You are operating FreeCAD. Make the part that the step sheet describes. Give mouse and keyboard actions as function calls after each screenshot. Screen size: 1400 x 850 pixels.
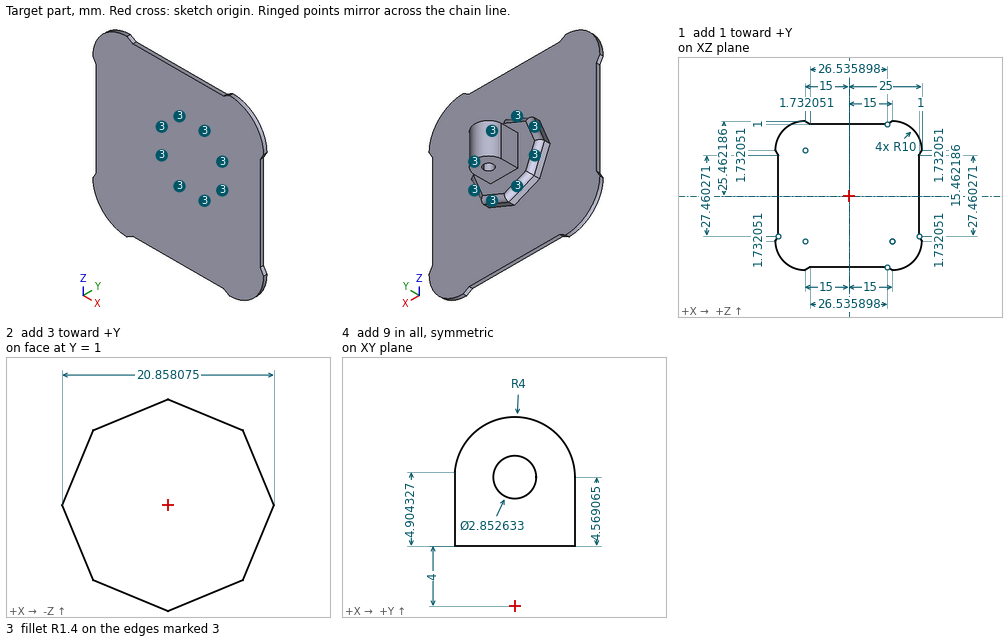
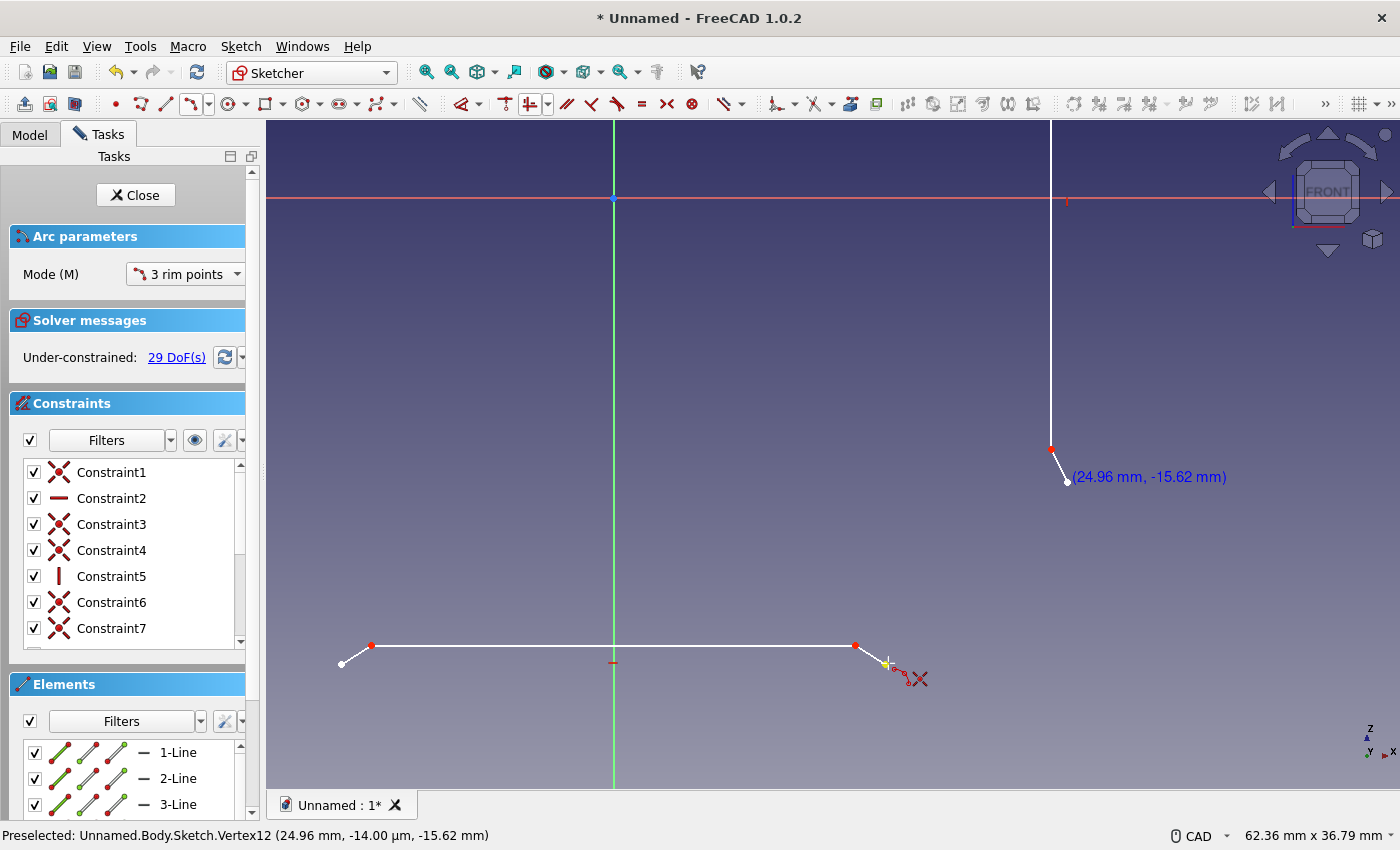
click(885, 665)
click(1015, 608)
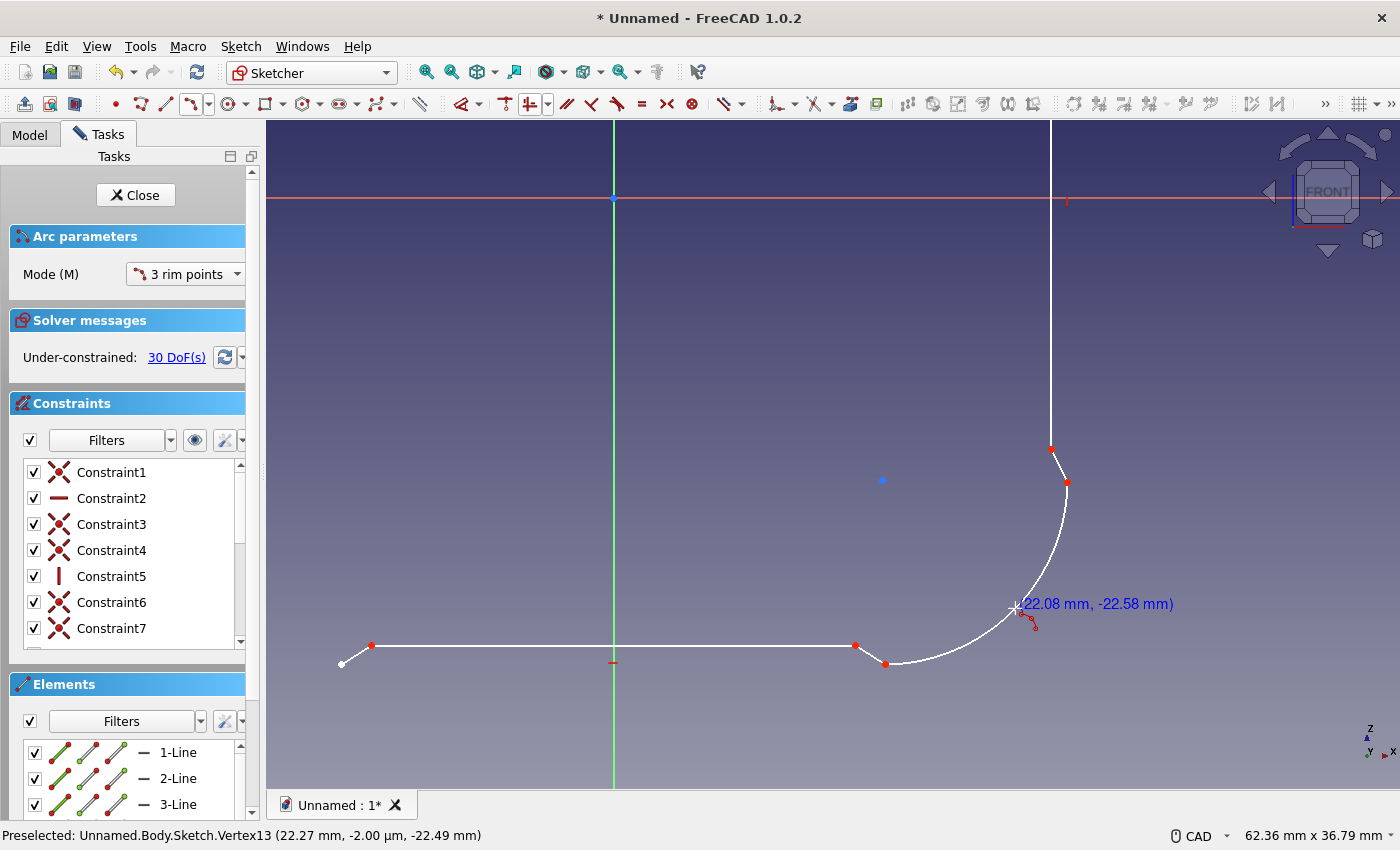
click(342, 665)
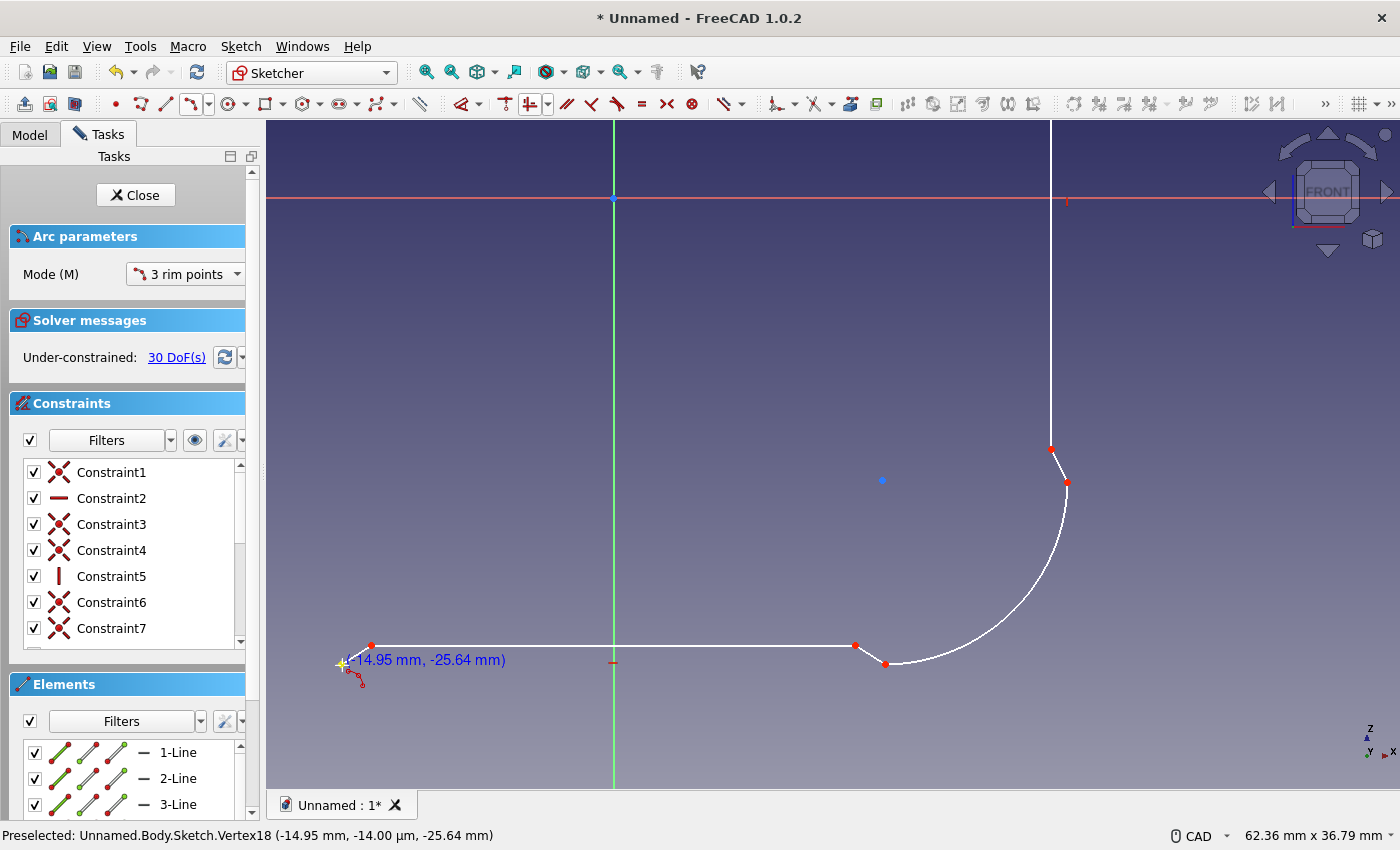
scroll(888, 663, down, 4)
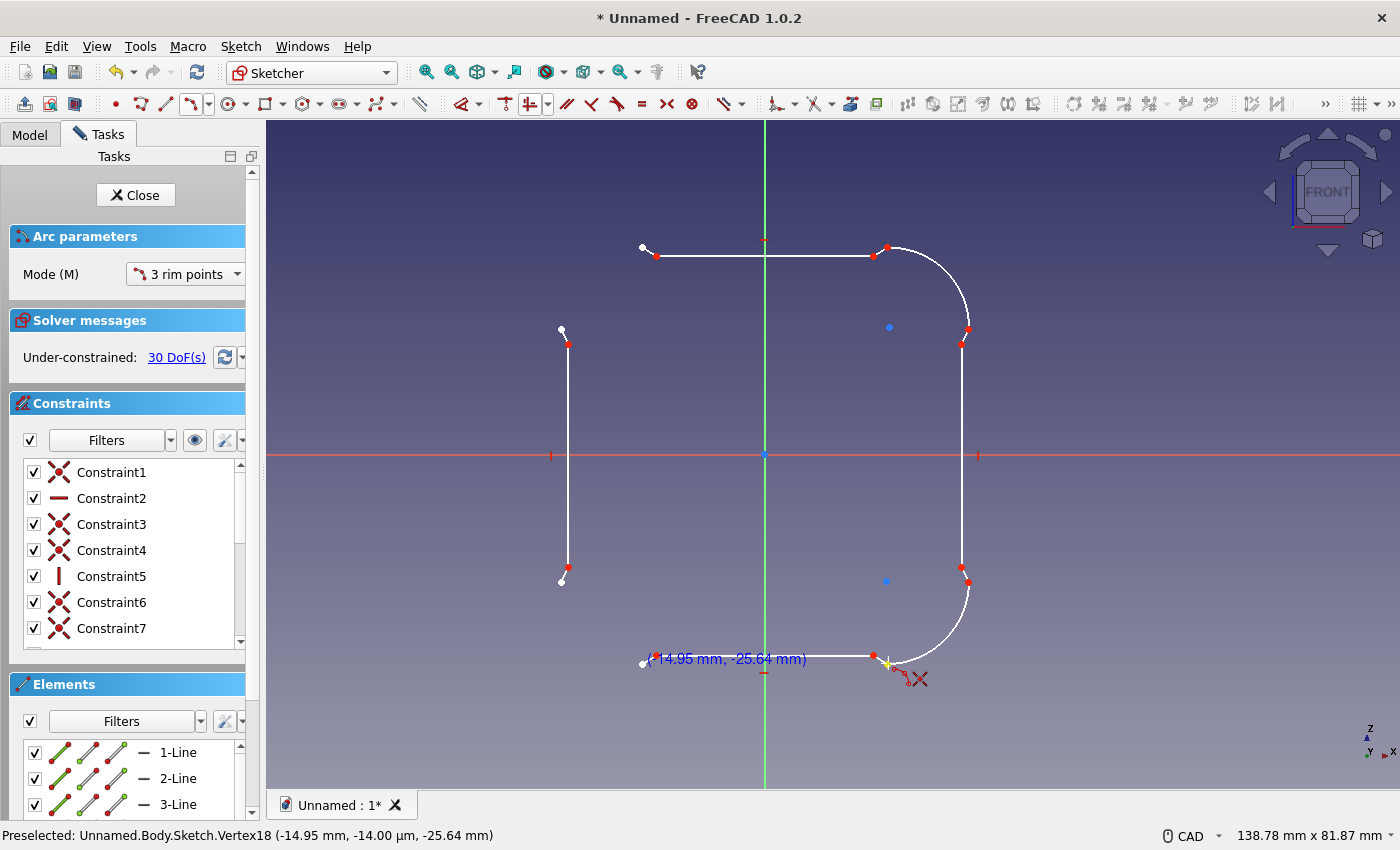
scroll(561, 581, up, 4)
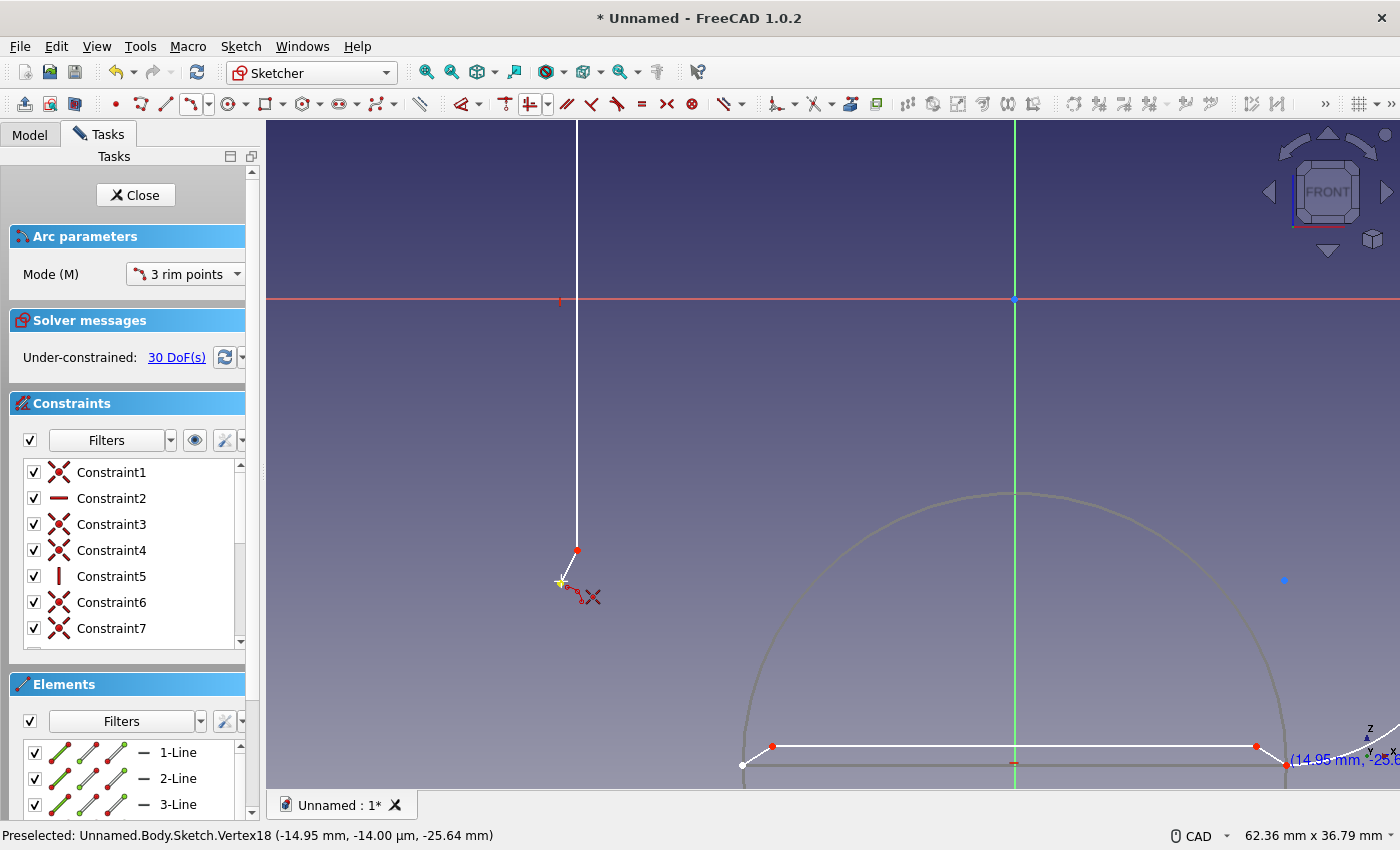
click(561, 583)
click(613, 709)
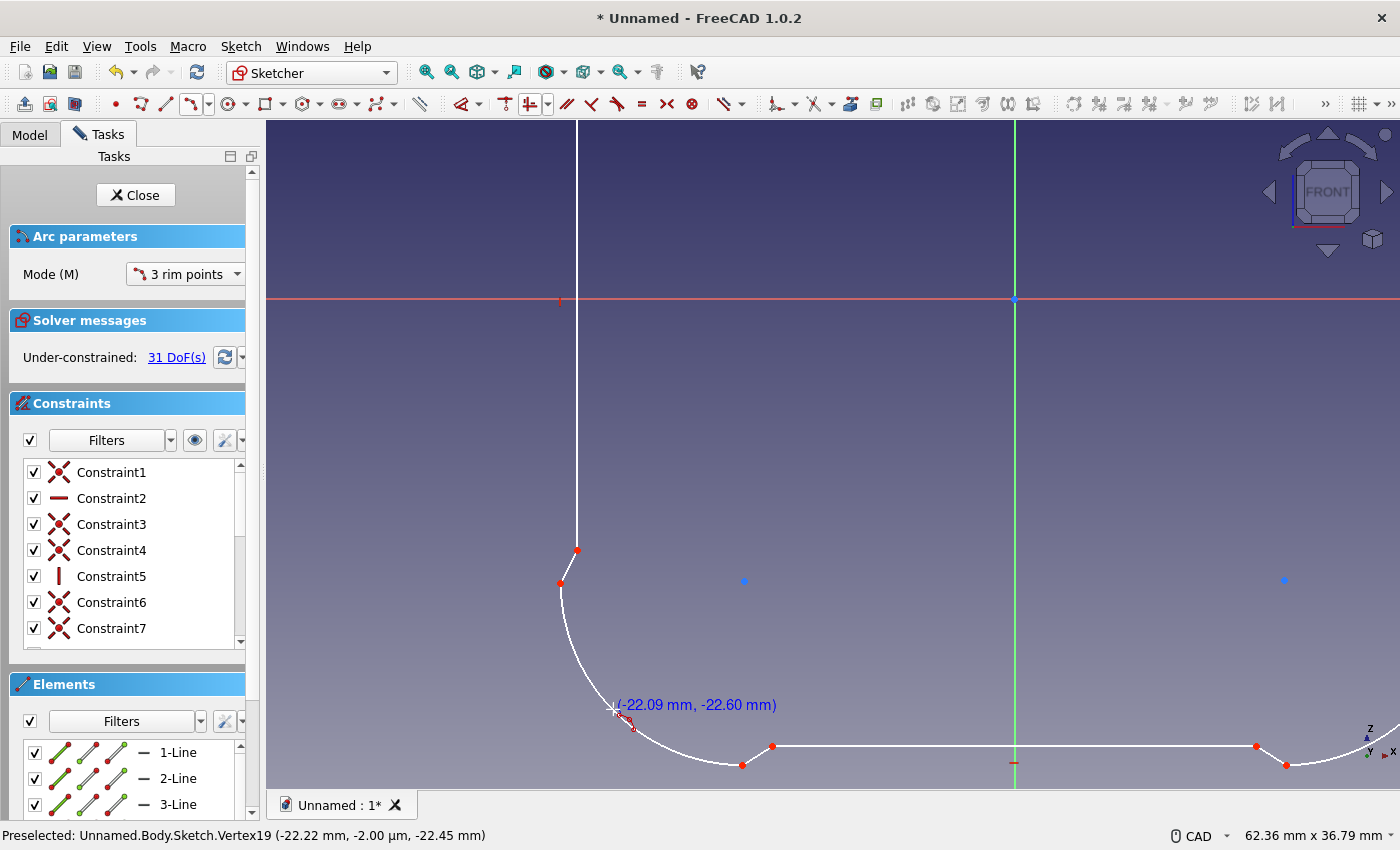
scroll(560, 581, down, 4)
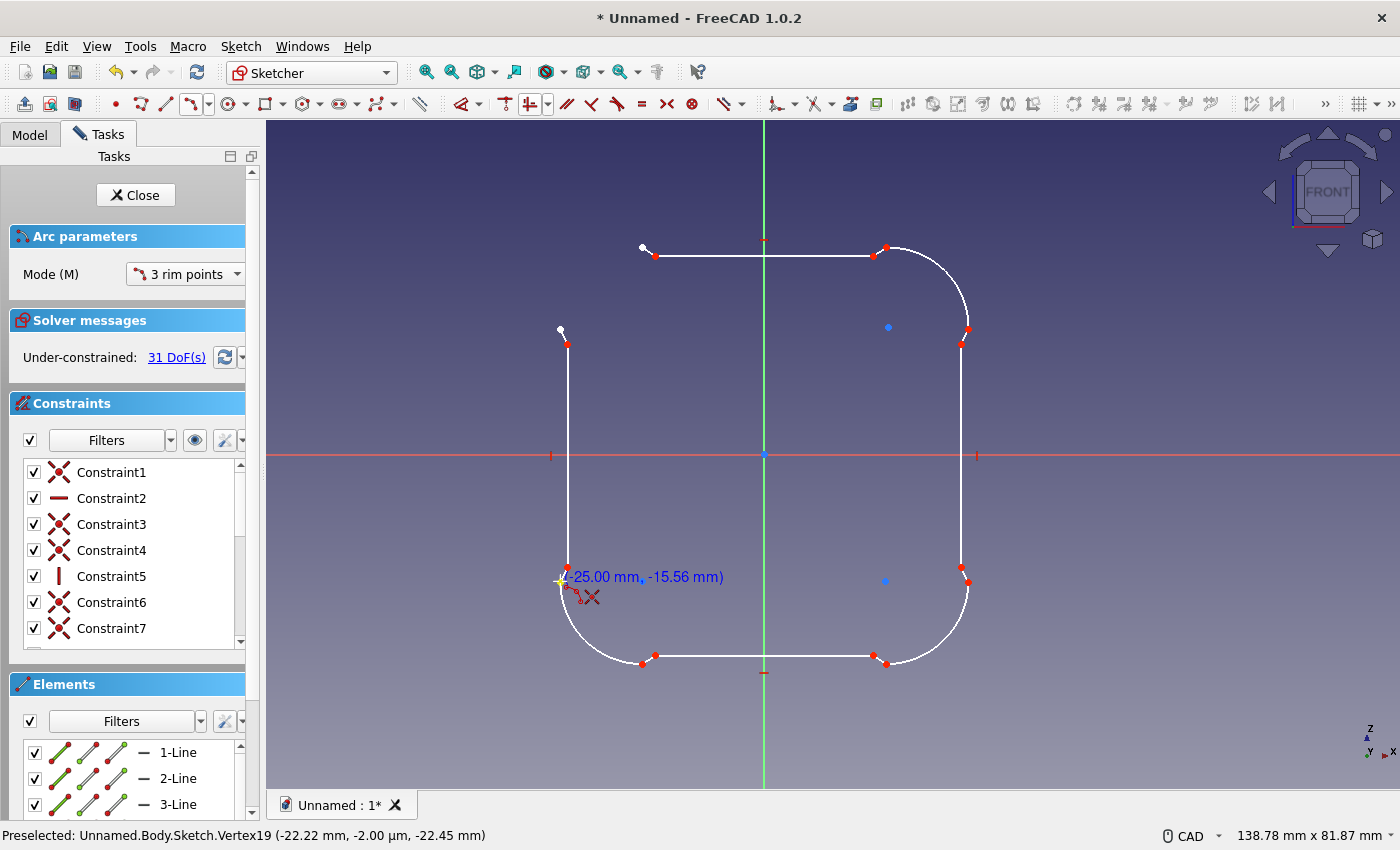
scroll(560, 328, up, 4)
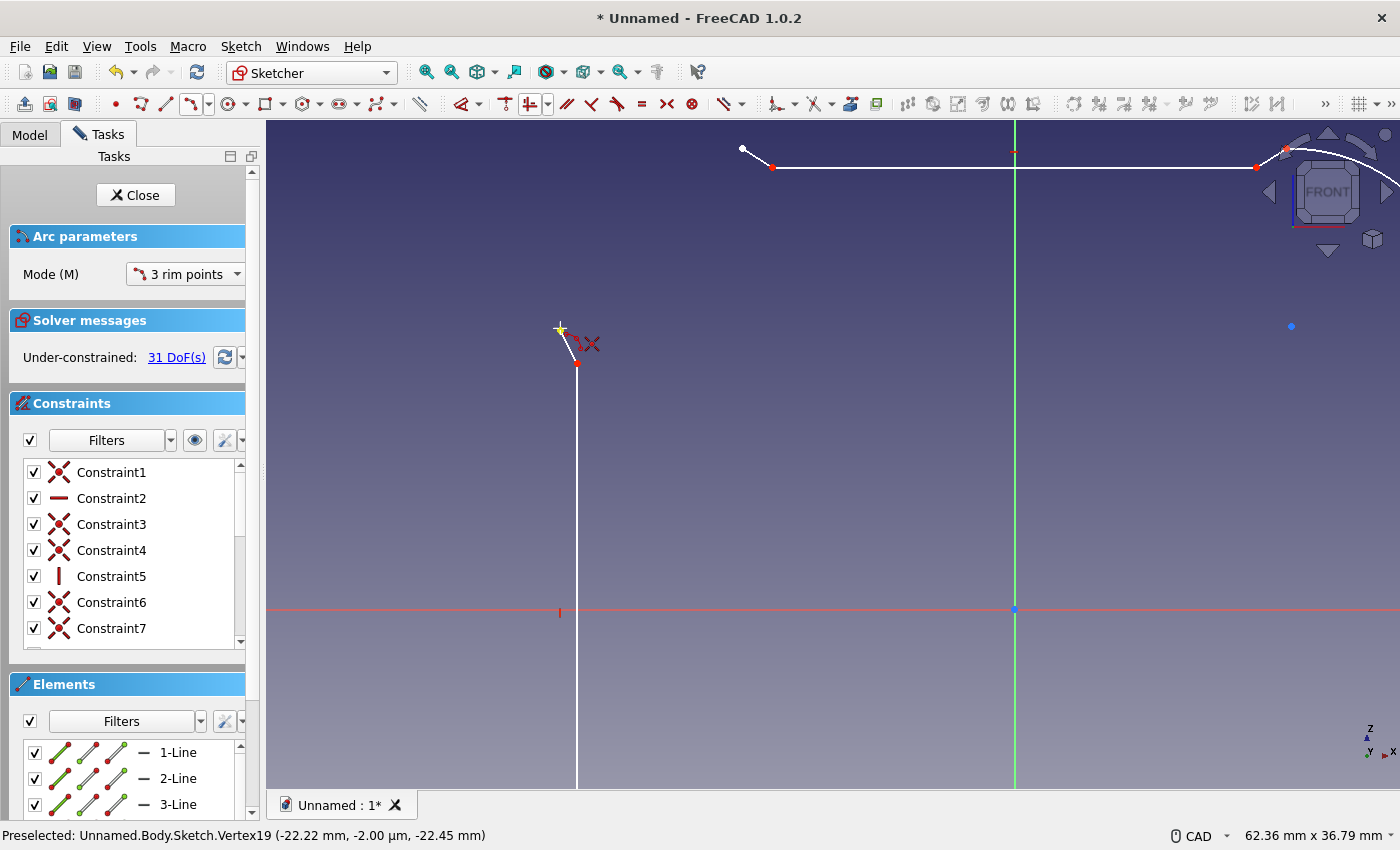
click(561, 331)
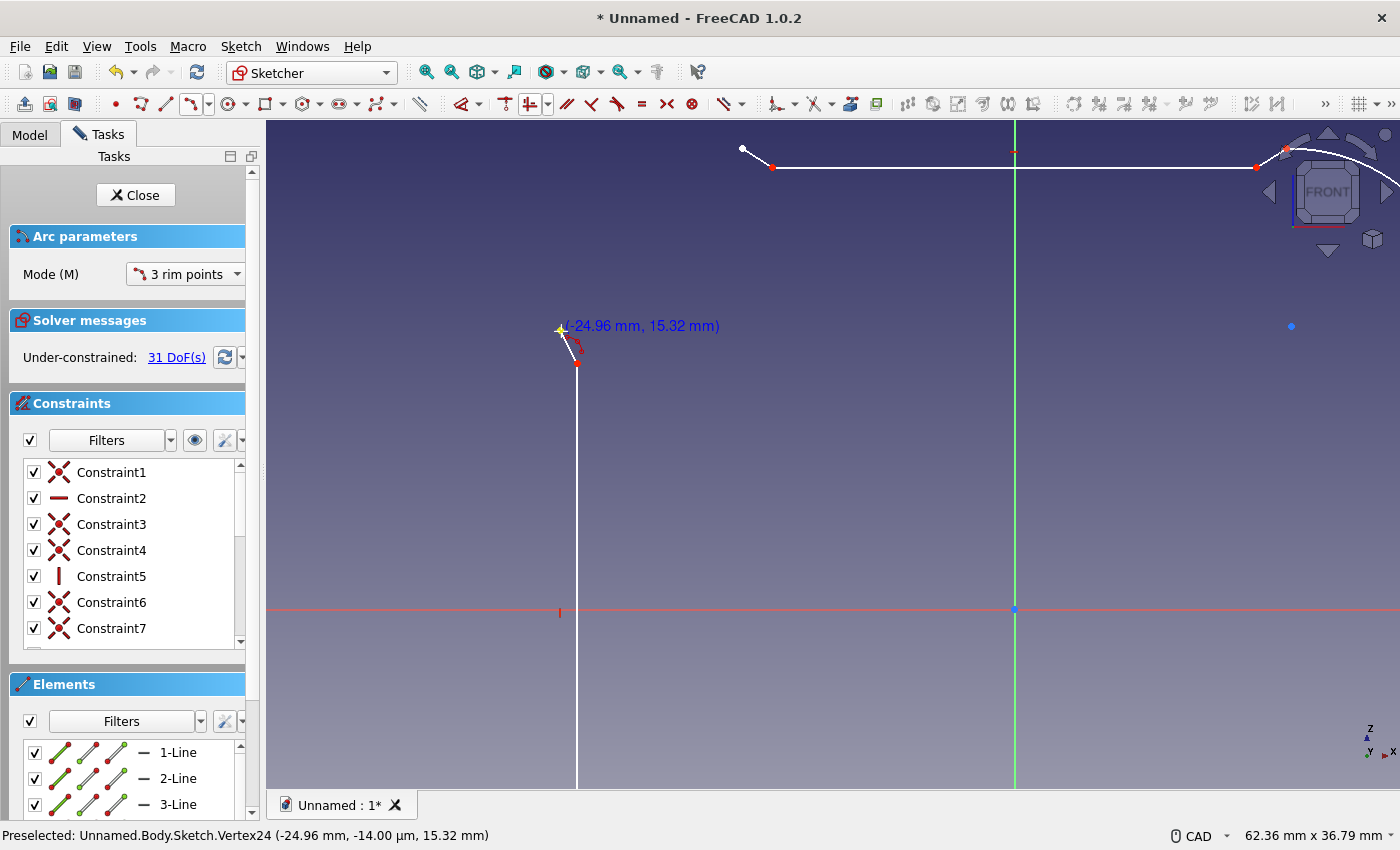
scroll(560, 328, down, 4)